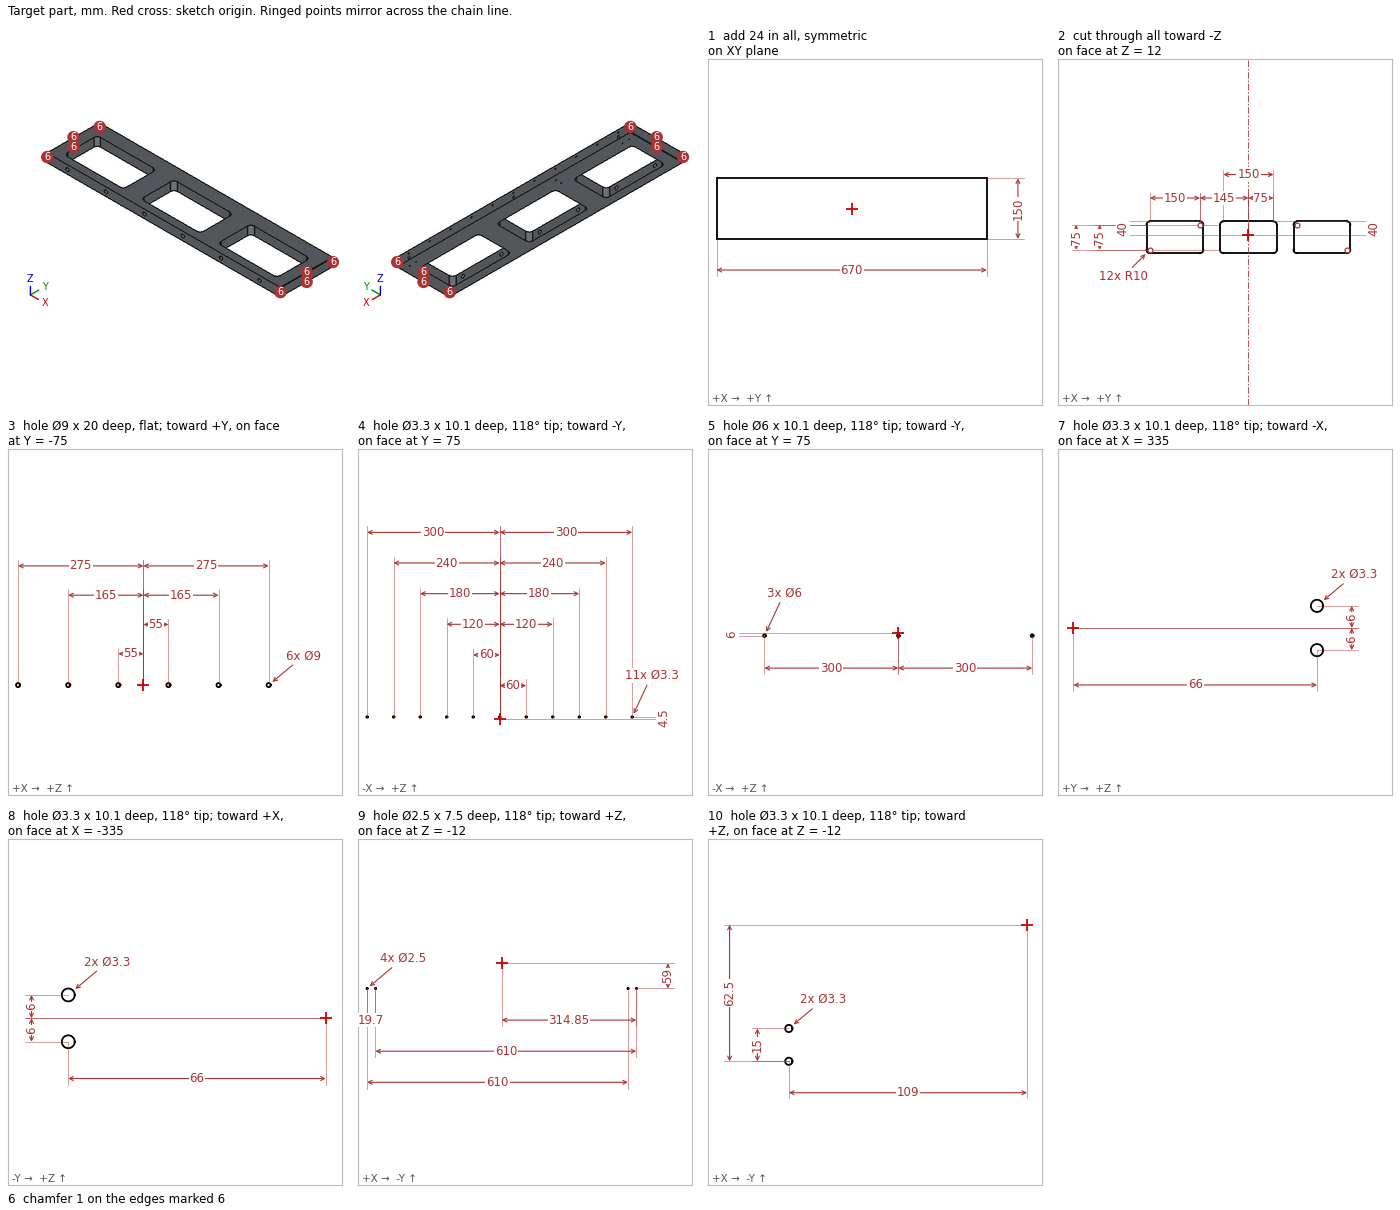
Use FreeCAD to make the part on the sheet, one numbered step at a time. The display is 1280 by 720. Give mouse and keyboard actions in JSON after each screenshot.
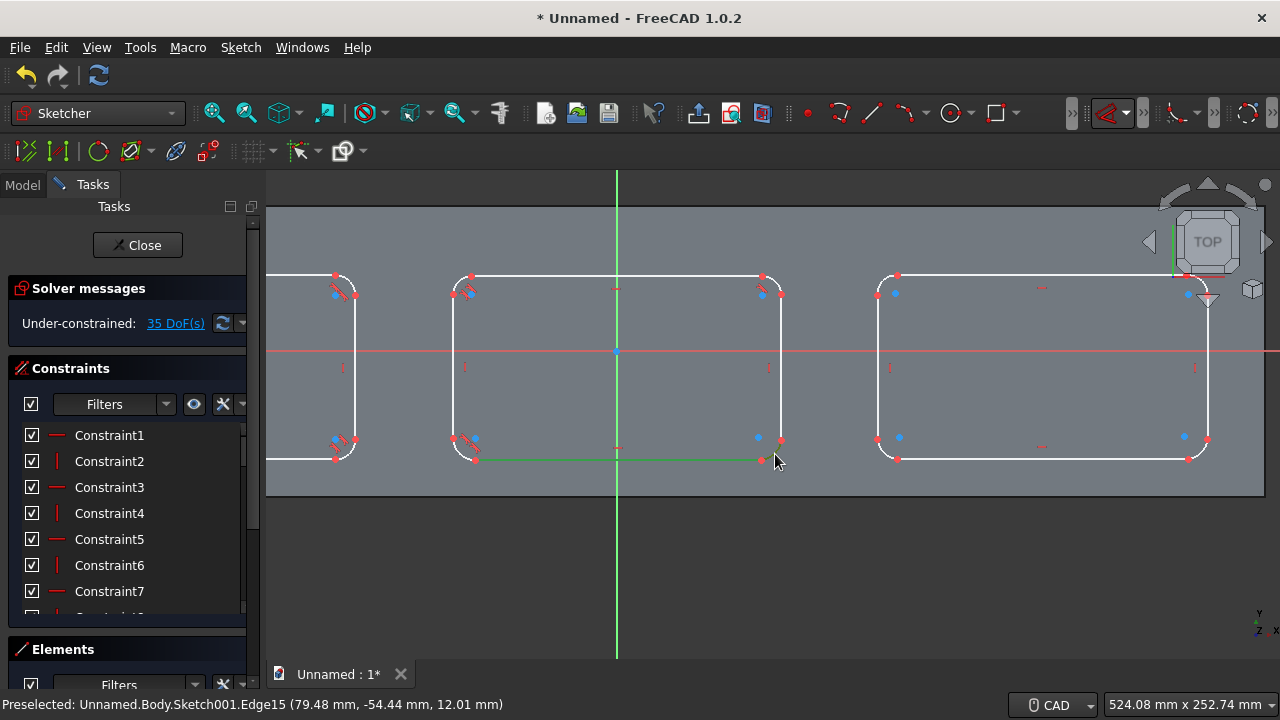
{"action": "key", "text": "t"}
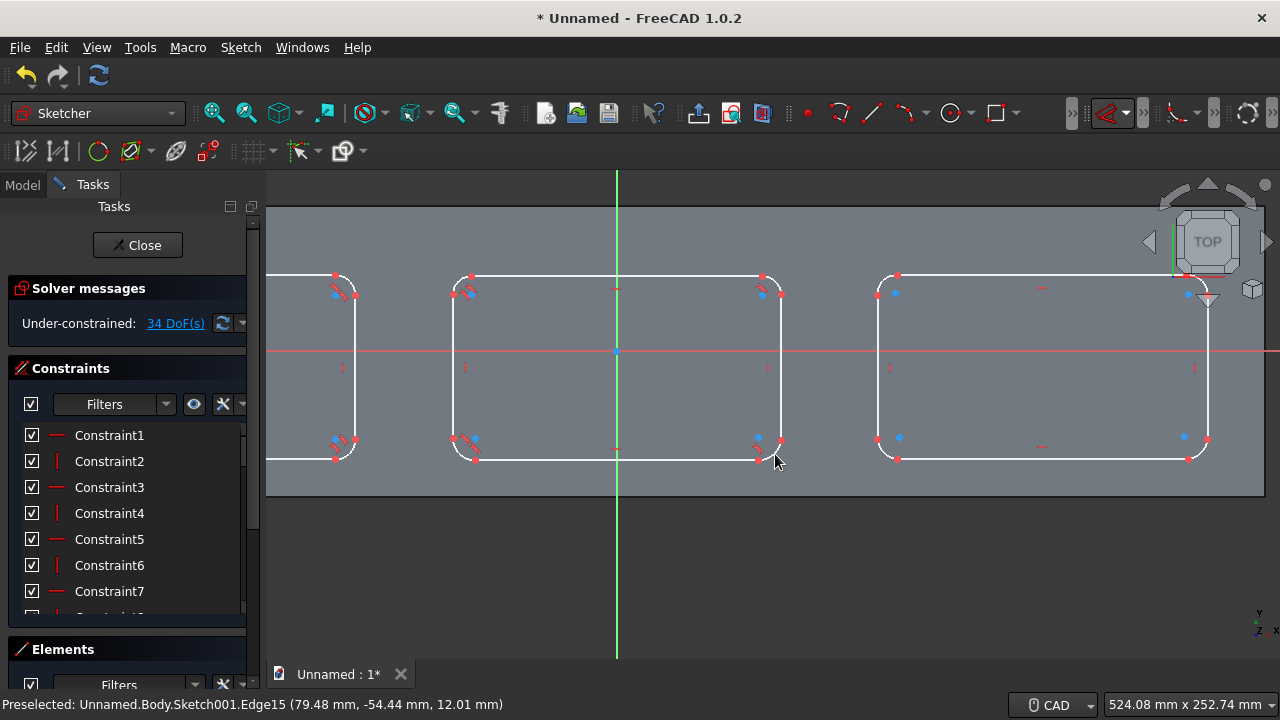
{"action": "left_click", "coordinate": [781, 397]}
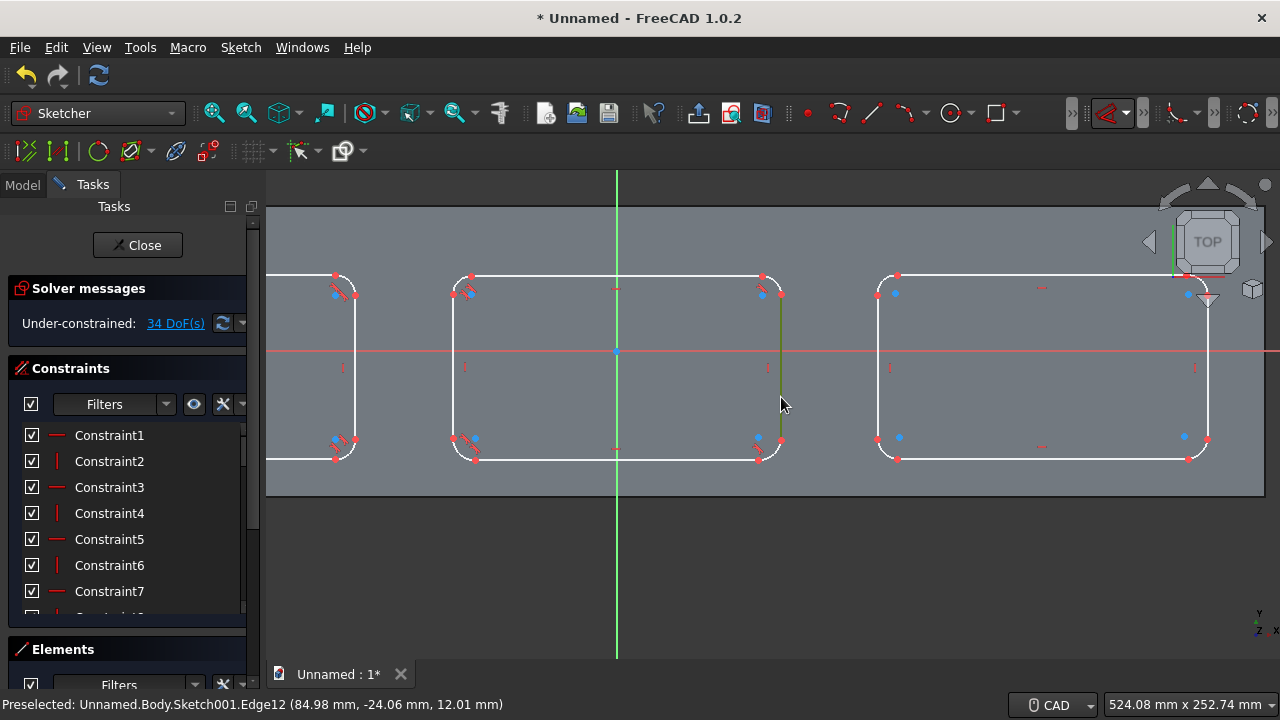
{"action": "scroll", "coordinate": [768, 458], "scroll_direction": "up", "scroll_amount": 2}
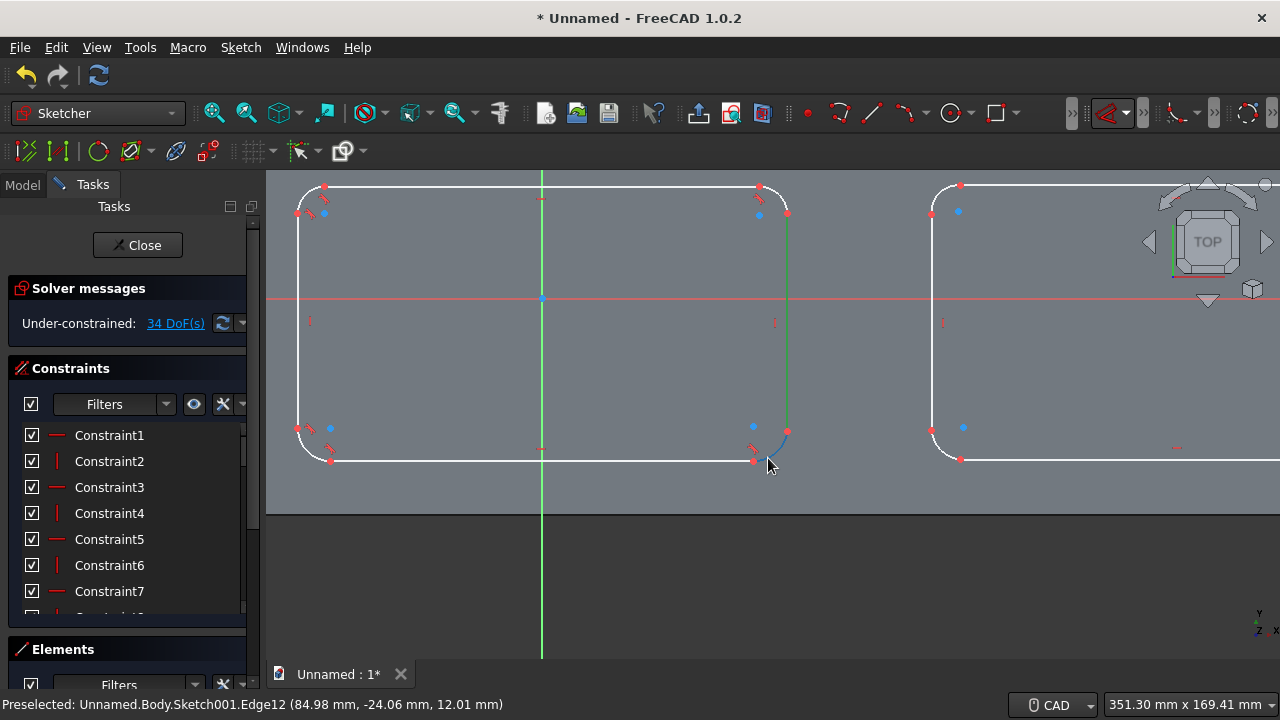
{"action": "left_click", "coordinate": [767, 458]}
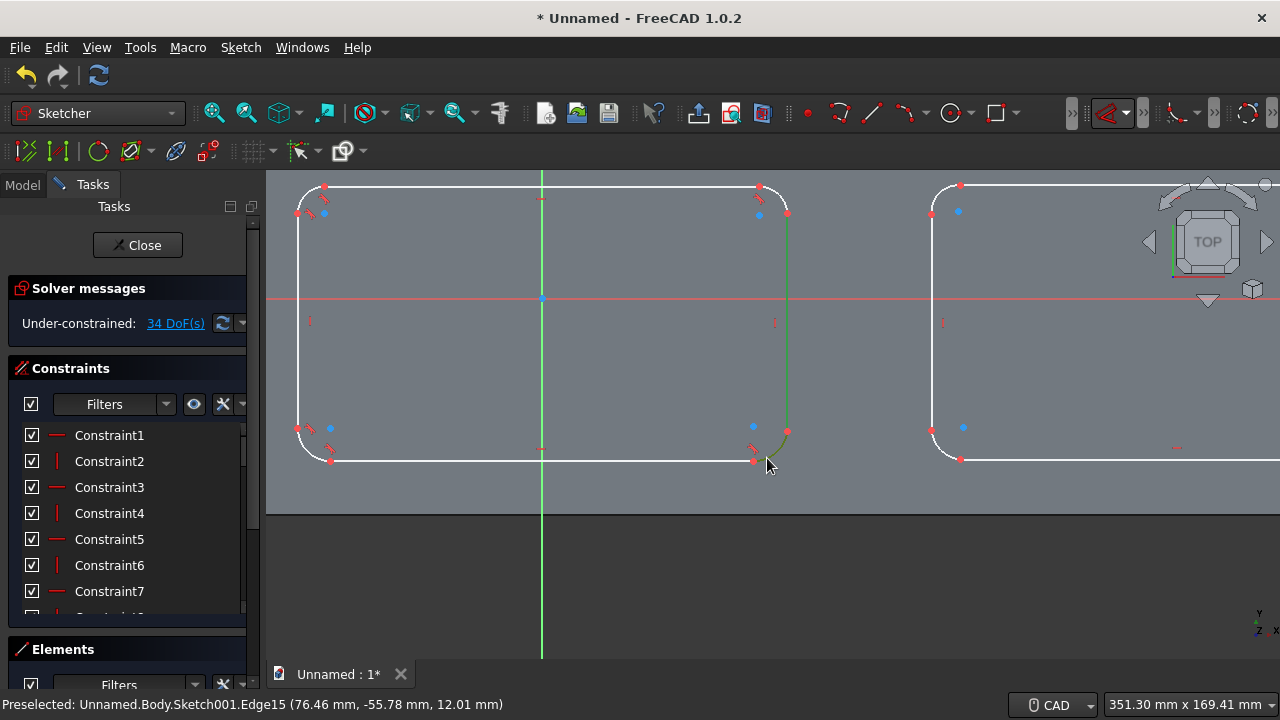
{"action": "key", "text": "t"}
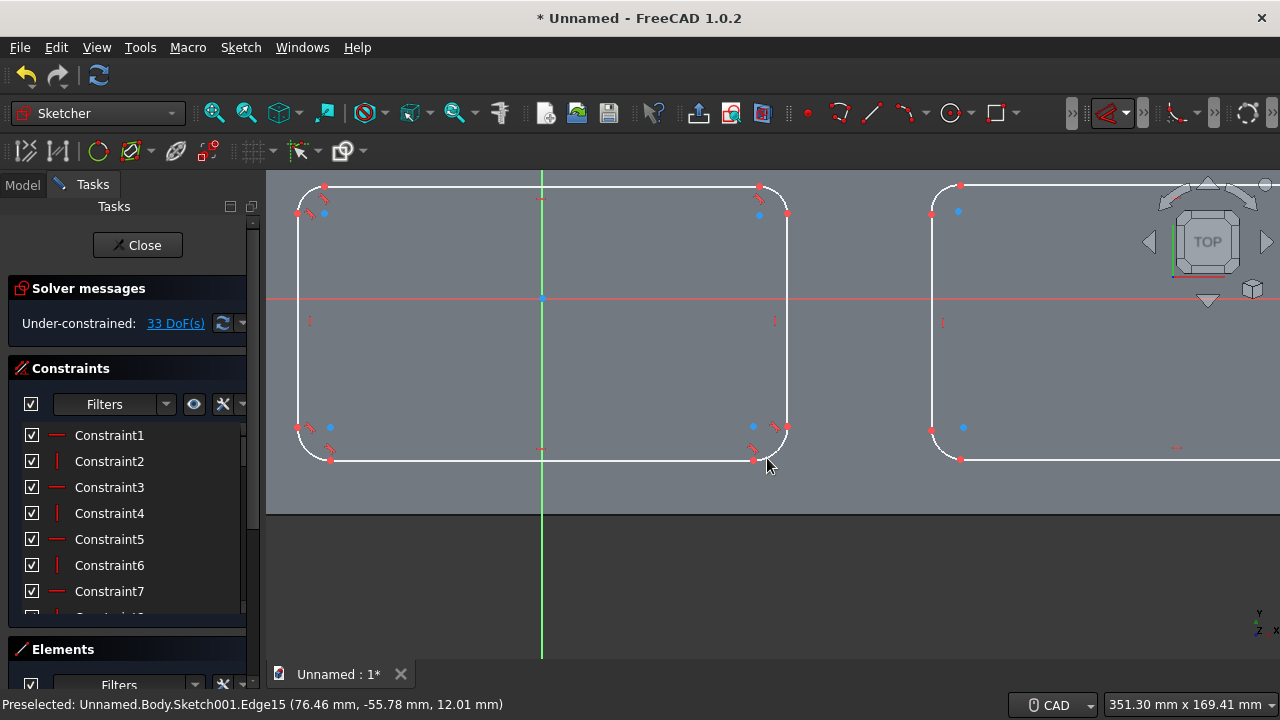
{"action": "scroll", "coordinate": [774, 455], "scroll_direction": "down", "scroll_amount": 6}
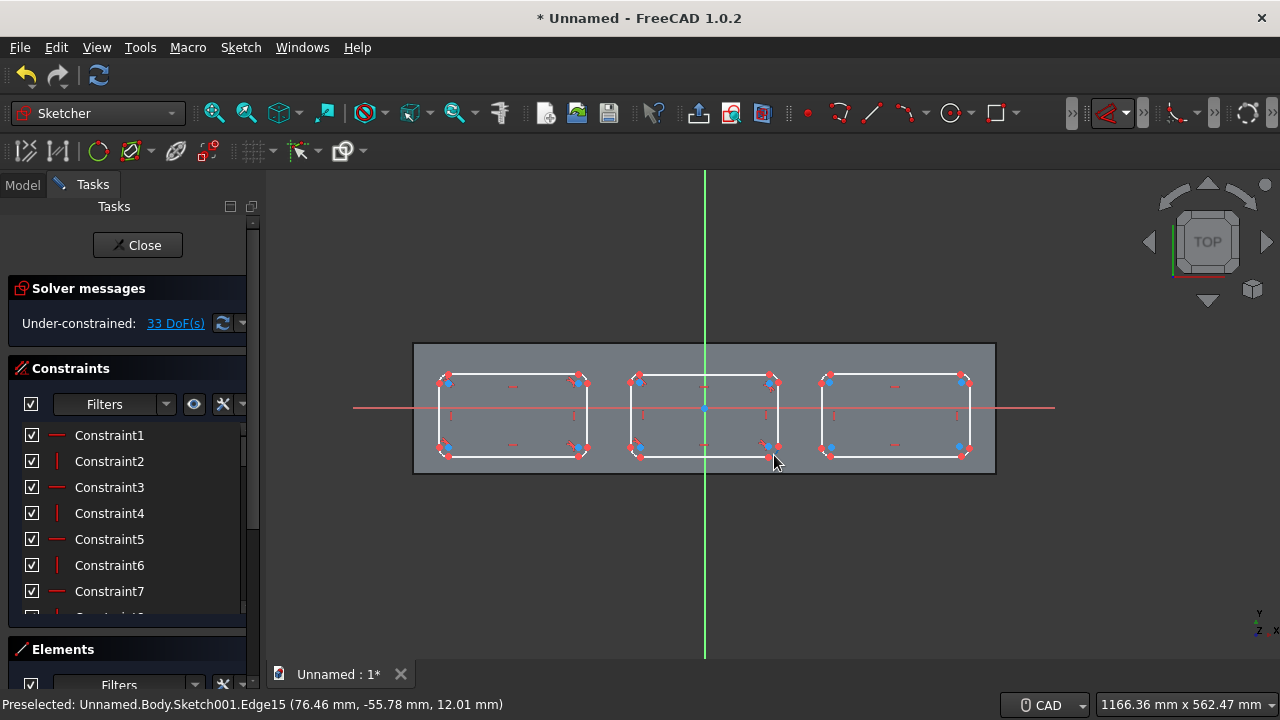
{"action": "left_click", "coordinate": [778, 428]}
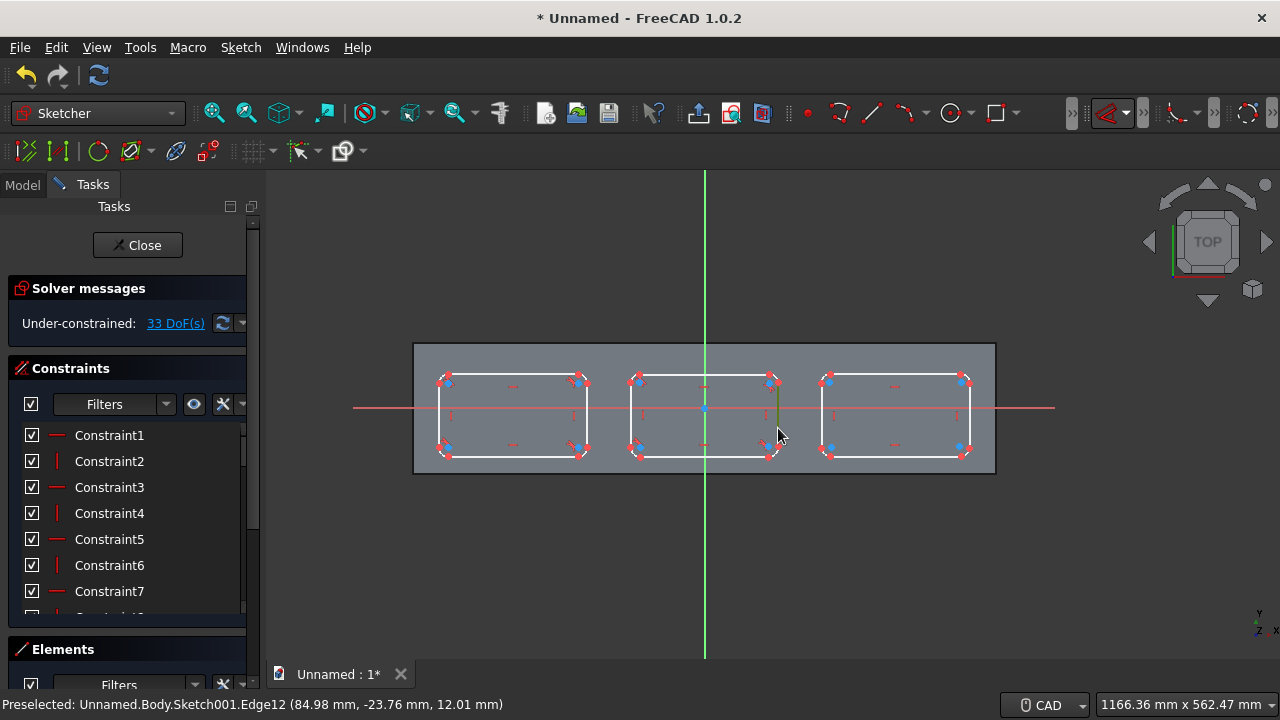
{"action": "scroll", "coordinate": [776, 377], "scroll_direction": "up", "scroll_amount": 4}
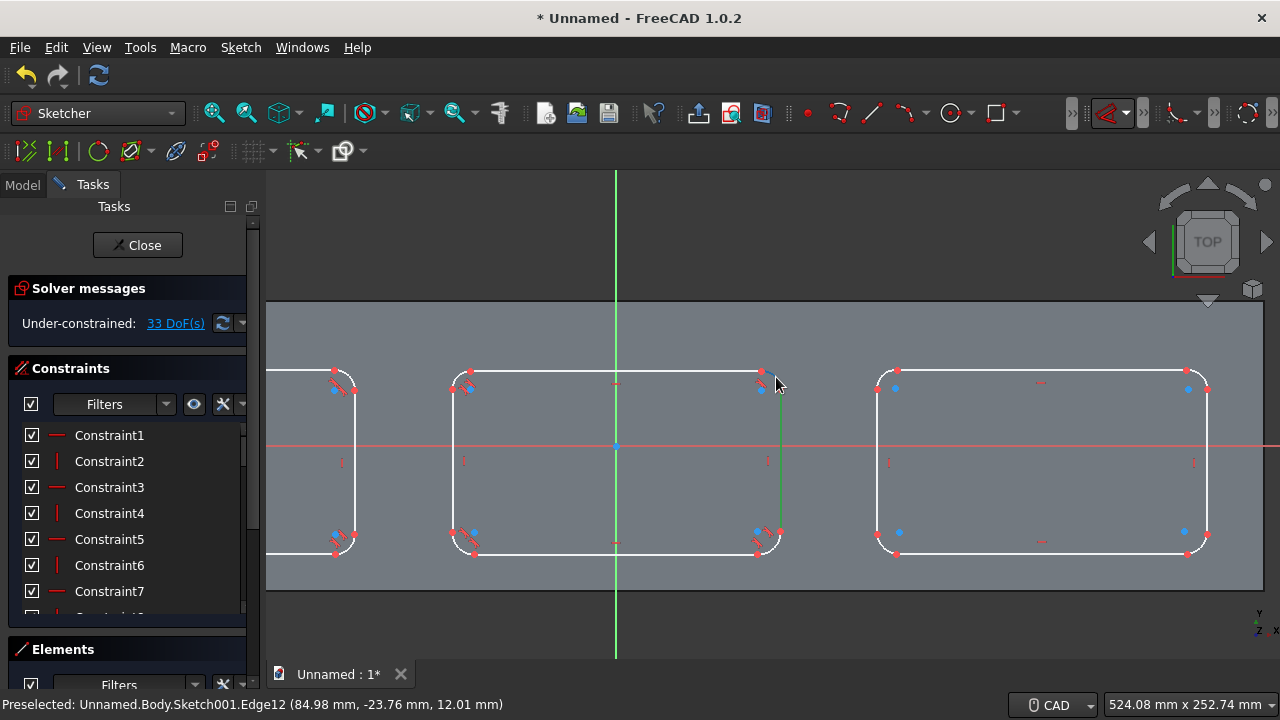
{"action": "left_click", "coordinate": [775, 376]}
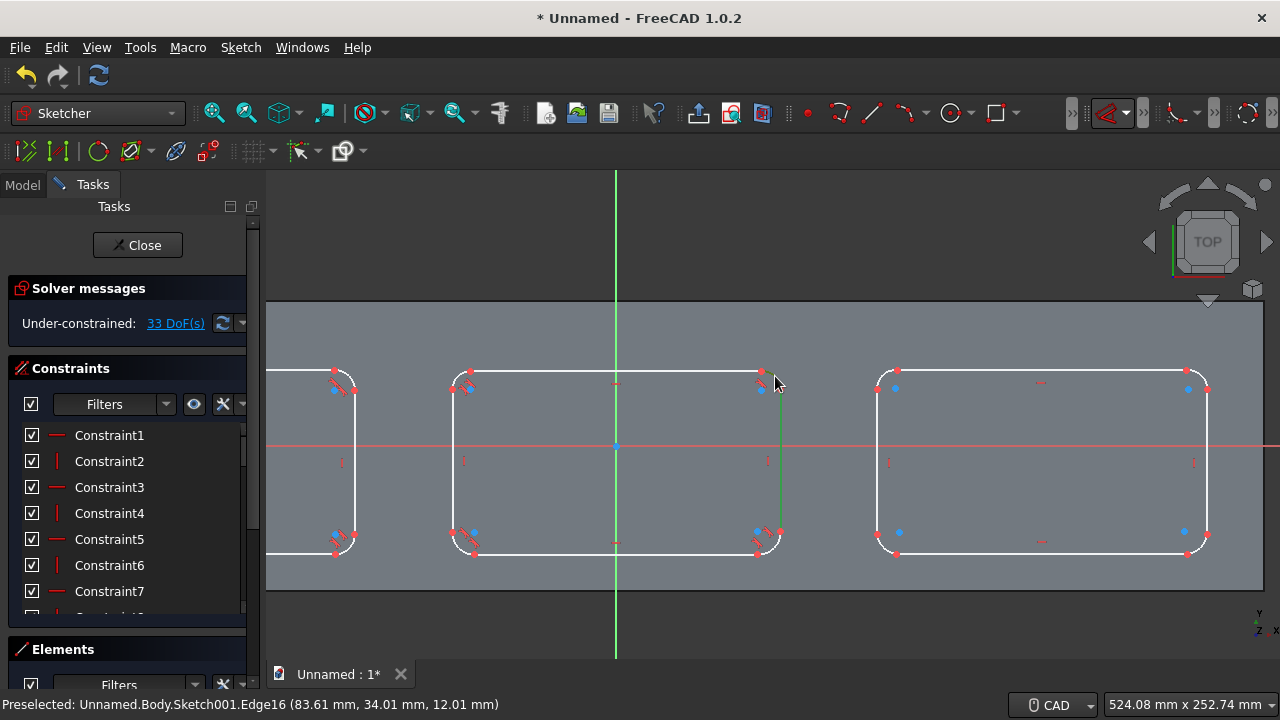
{"action": "key", "text": "t"}